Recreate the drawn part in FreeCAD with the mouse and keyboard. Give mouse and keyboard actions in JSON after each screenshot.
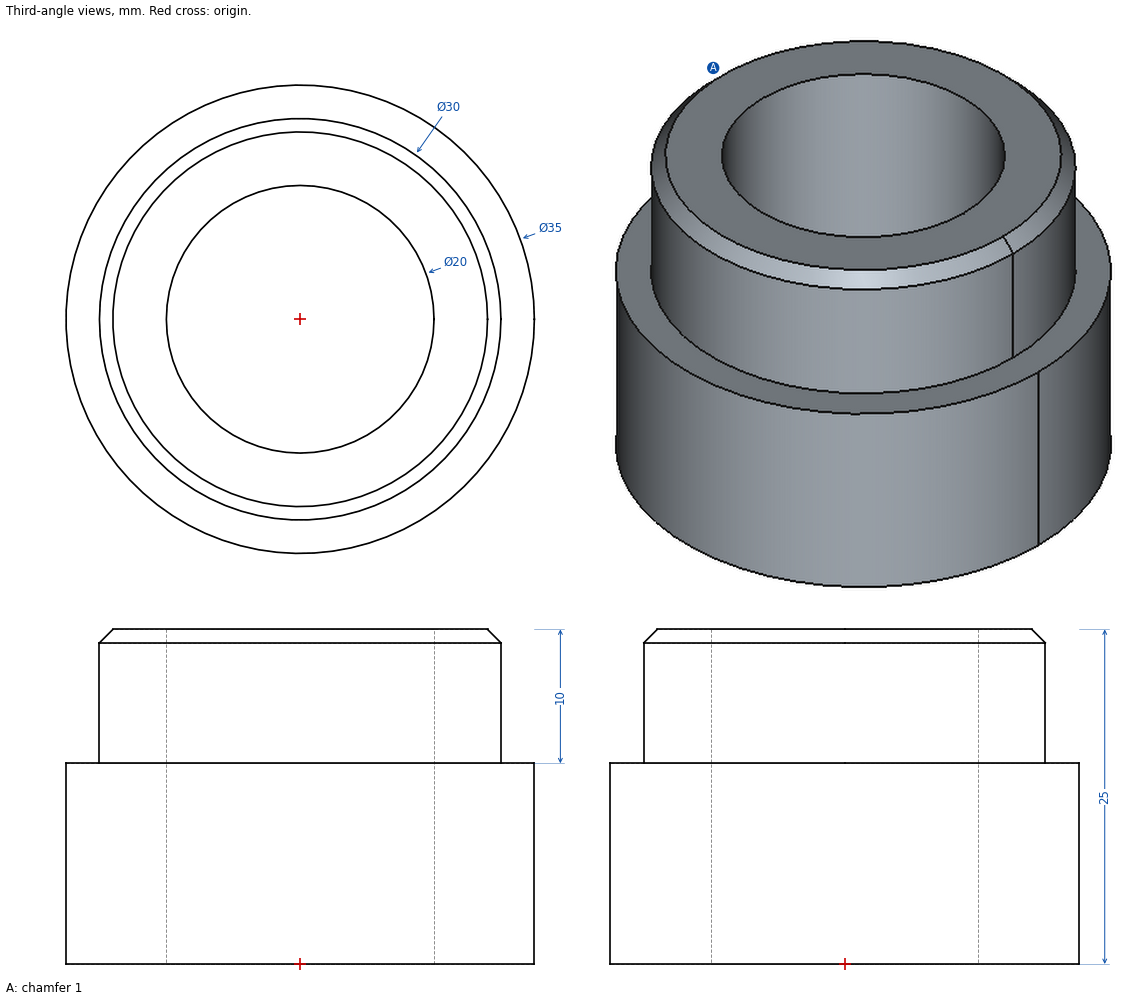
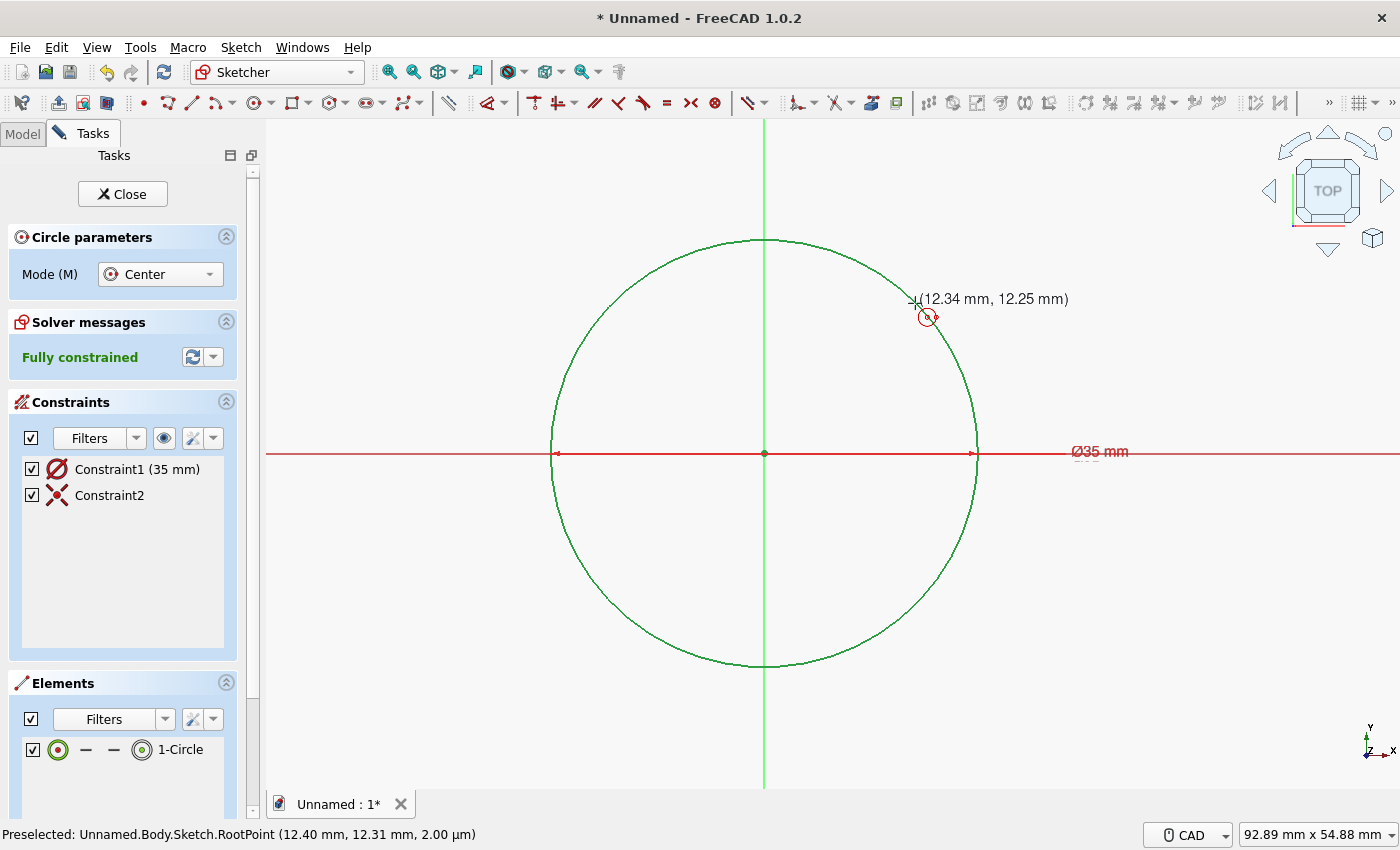
{"action": "left_click", "coordinate": [764, 454]}
{"action": "mouse_move", "coordinate": [851, 367]}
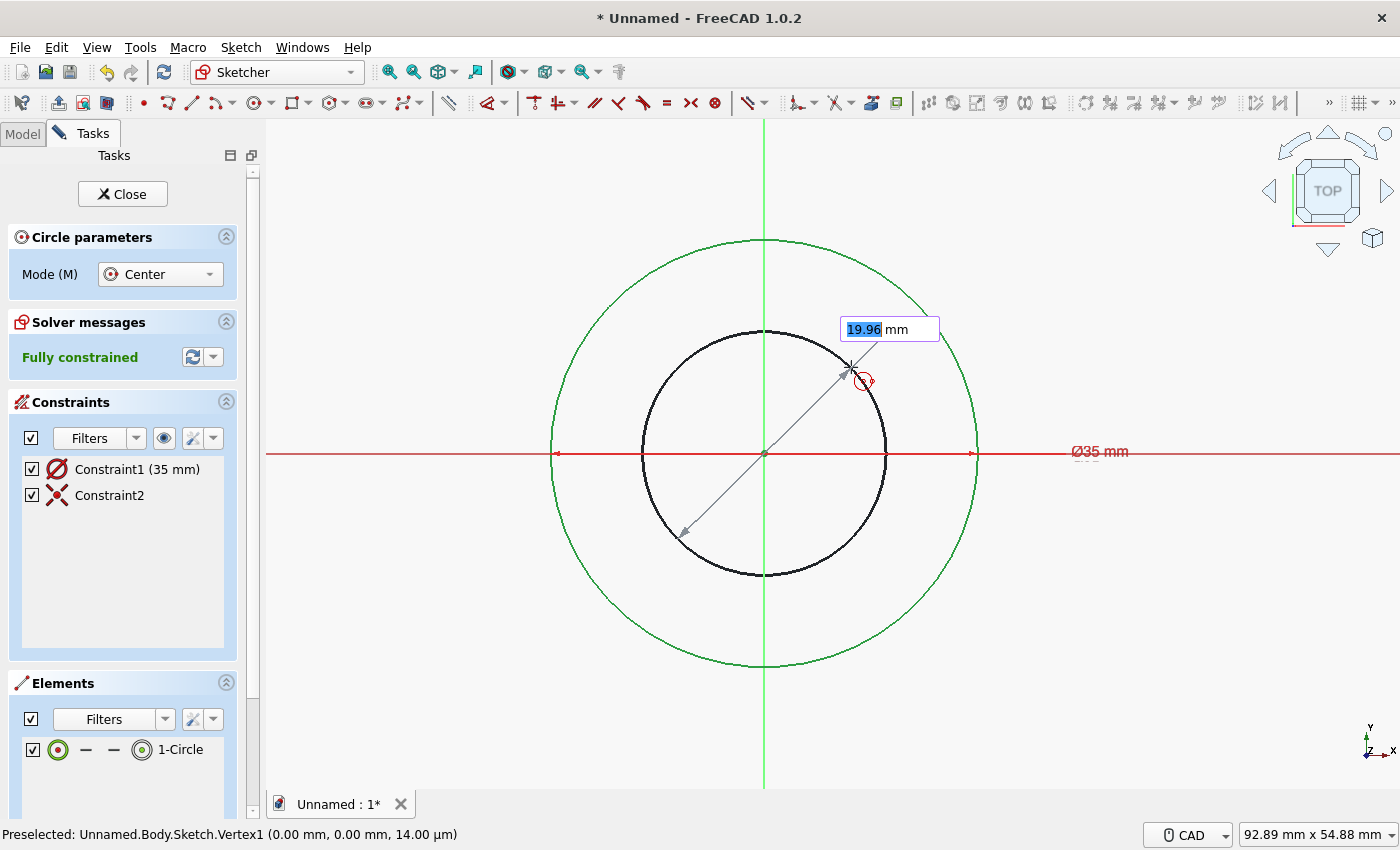
{"action": "type", "text": "20"}
{"action": "key", "text": "Return"}
{"action": "key", "text": "Escape"}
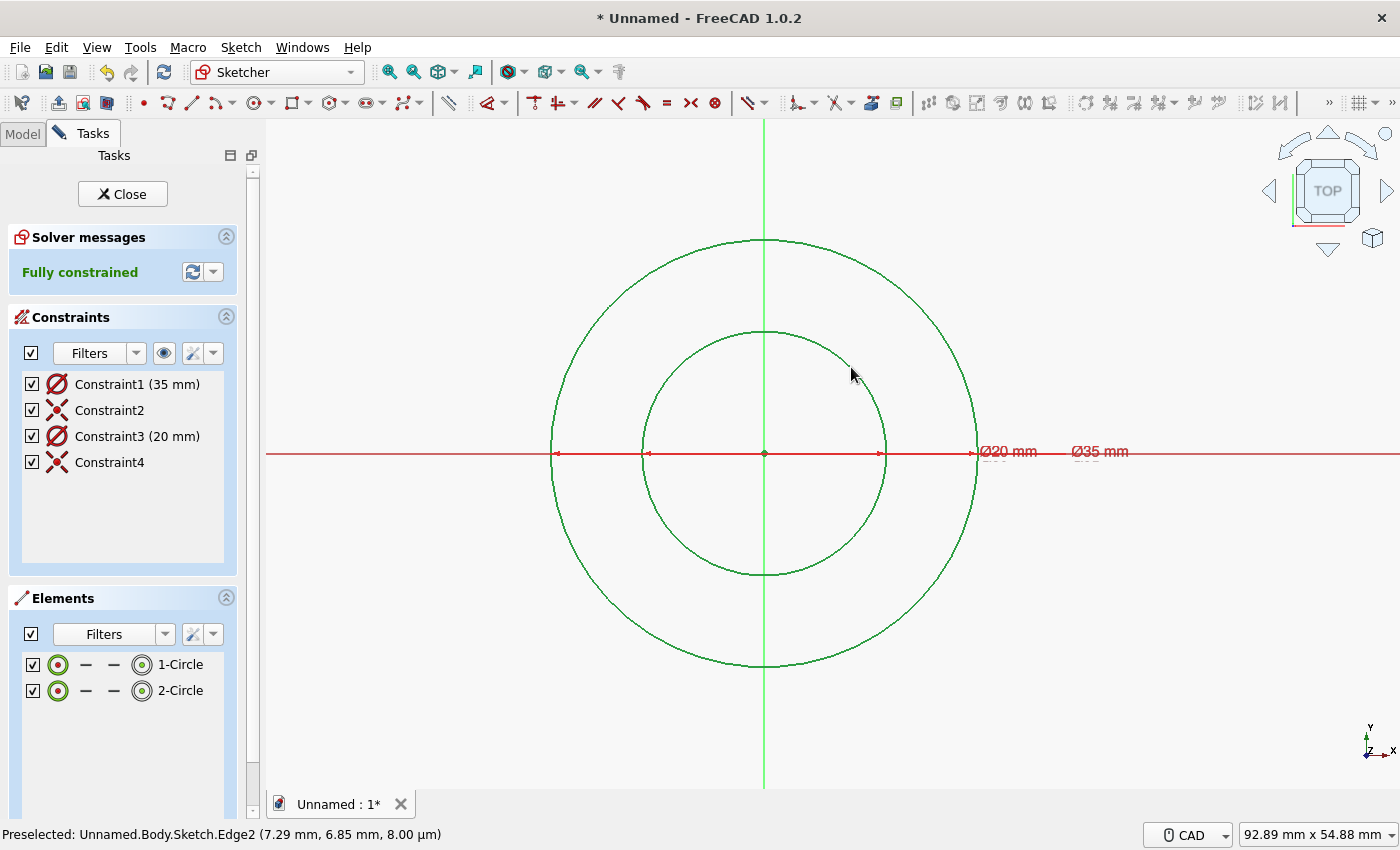
{"action": "left_click", "coordinate": [123, 194]}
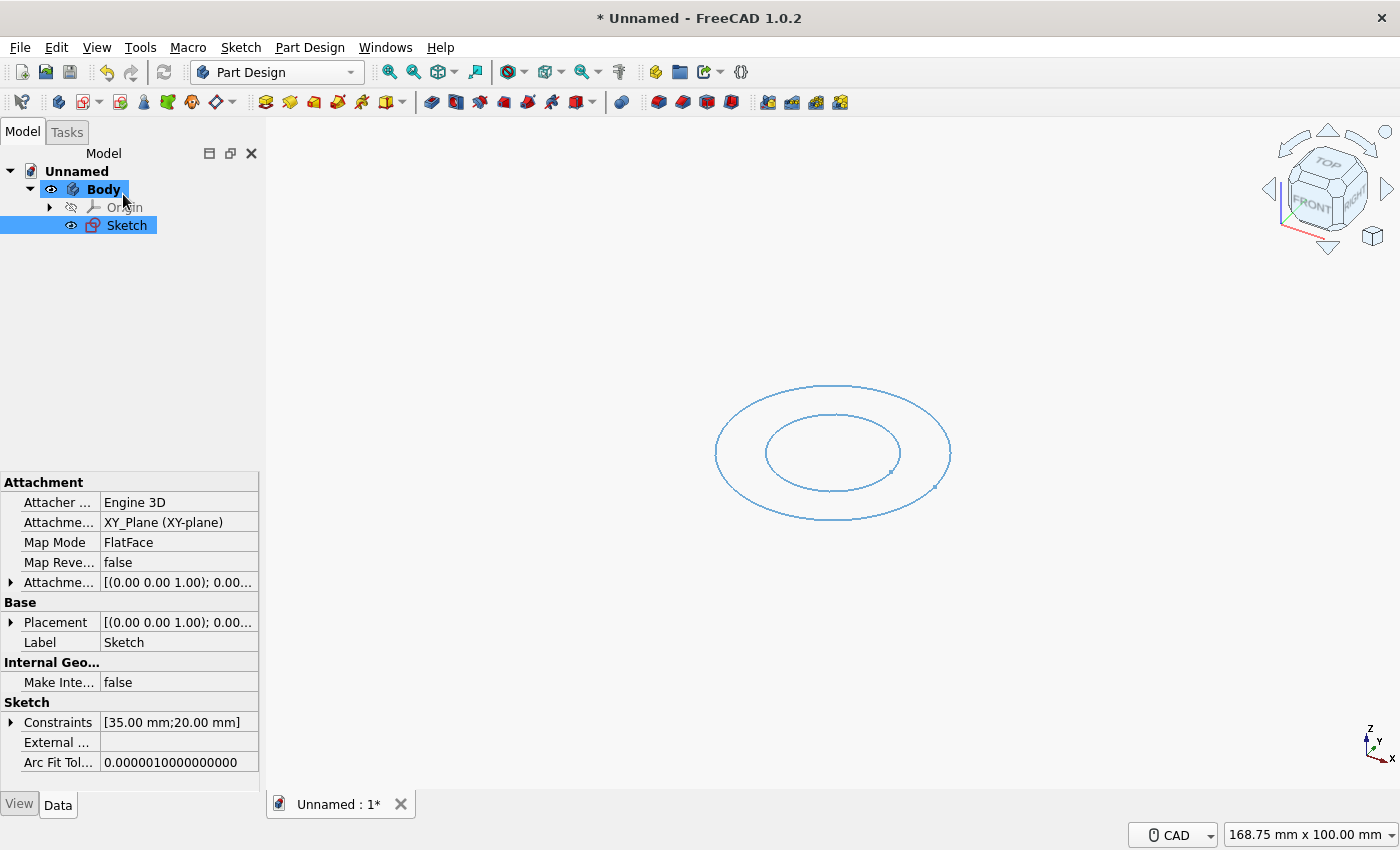
{"action": "left_click", "coordinate": [266, 102]}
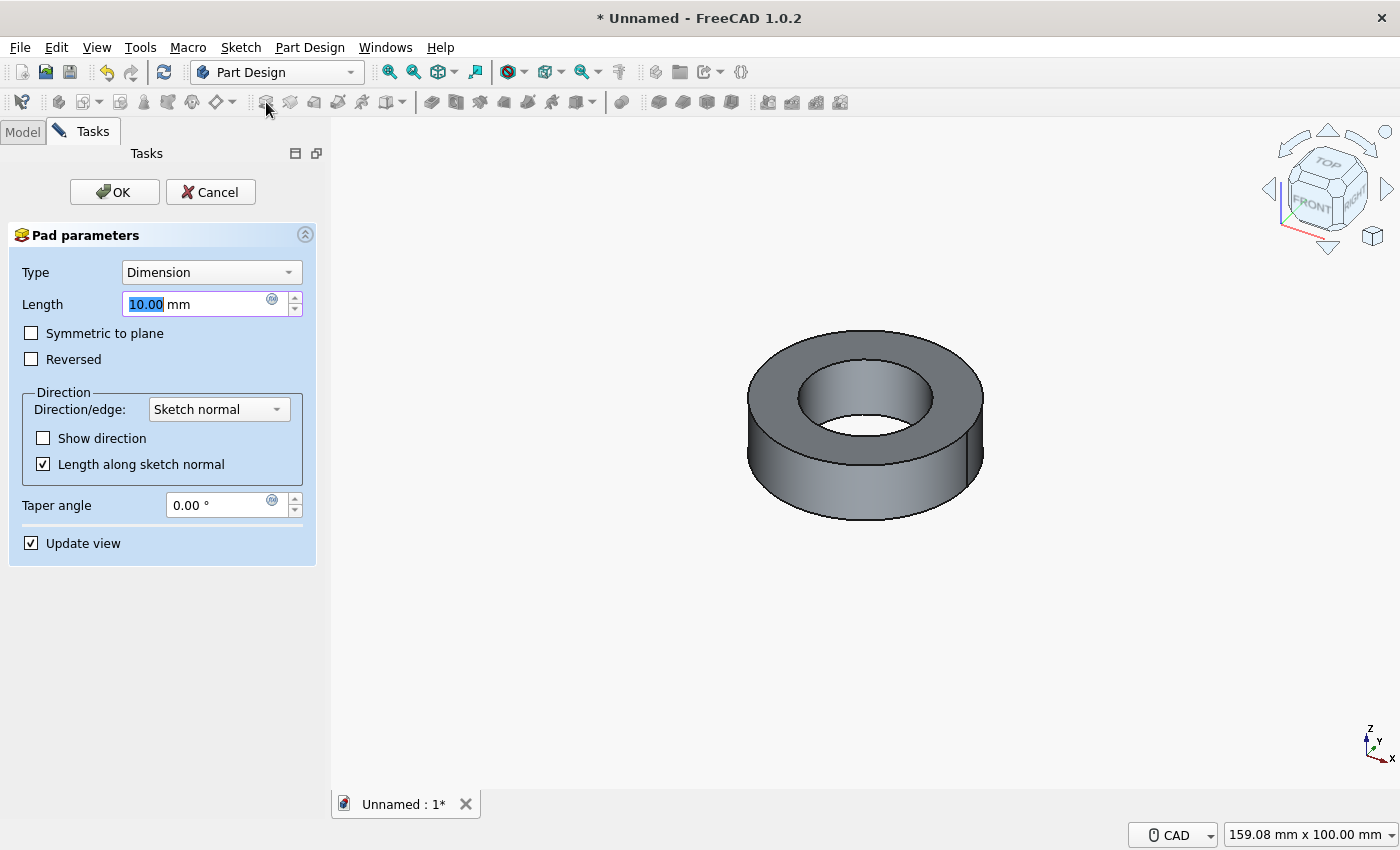
{"action": "type", "text": "25"}
{"action": "key", "text": "Tab"}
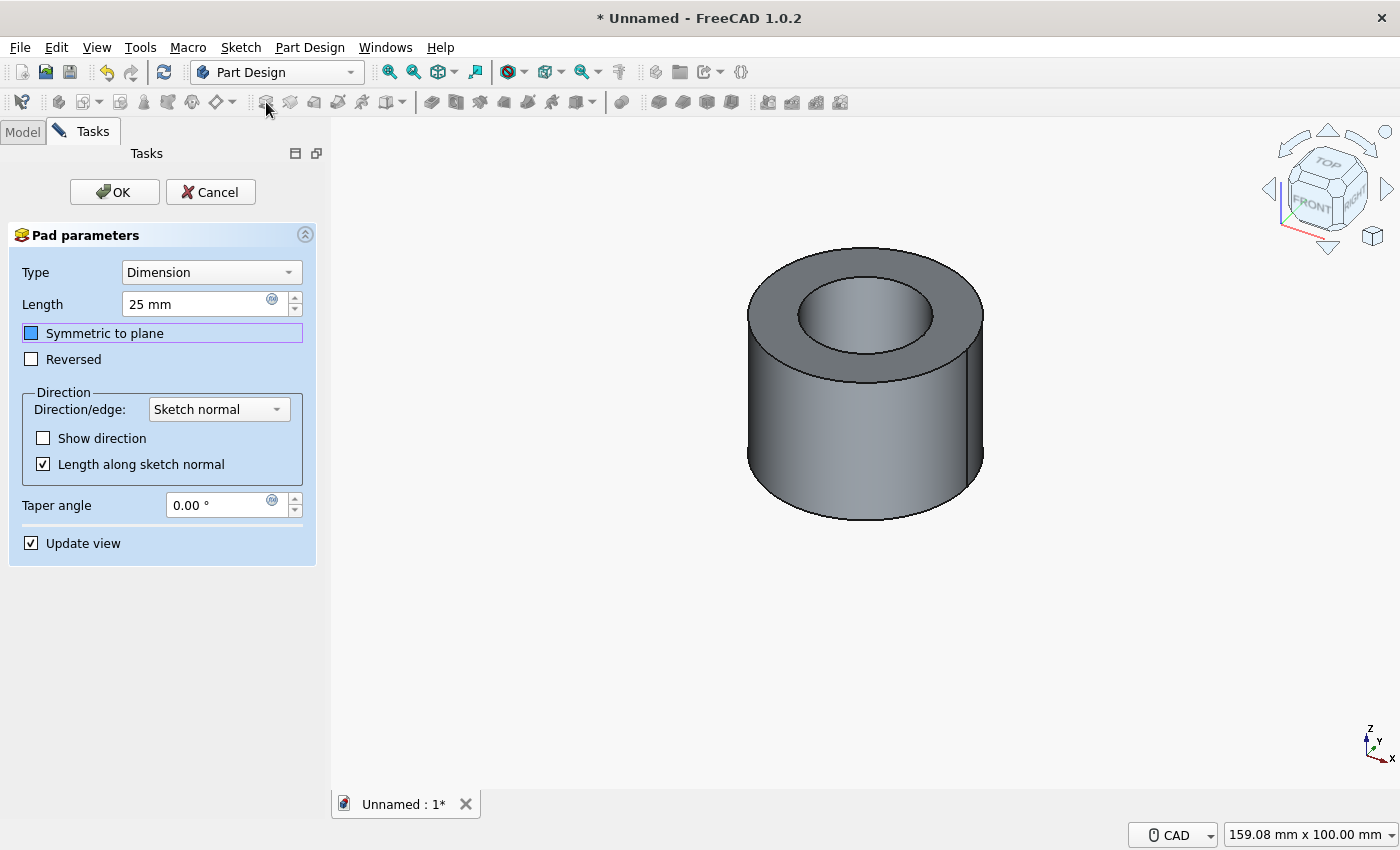
{"action": "left_click", "coordinate": [115, 192]}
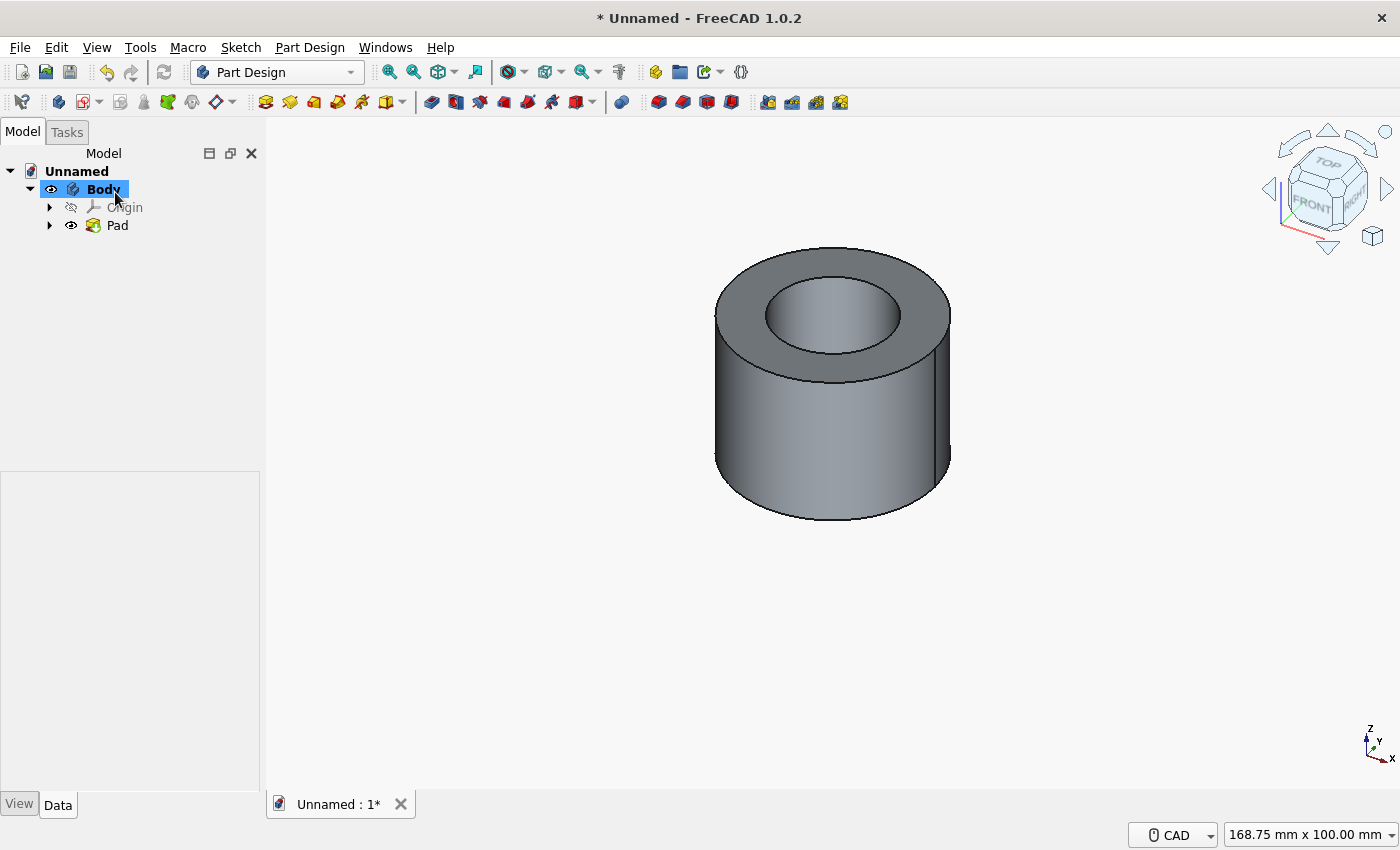
{"action": "left_click", "coordinate": [50, 207]}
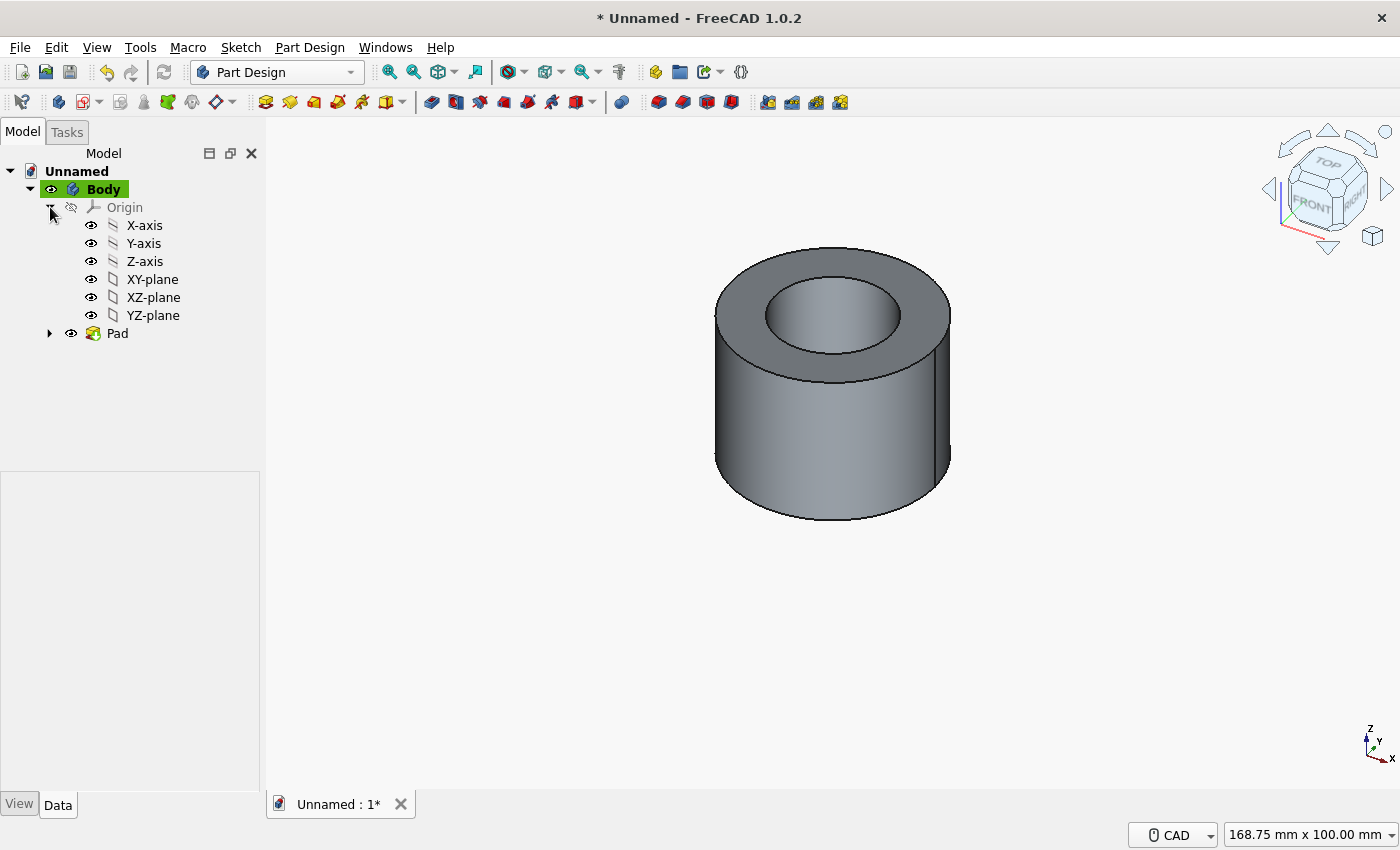
{"action": "left_click", "coordinate": [136, 279]}